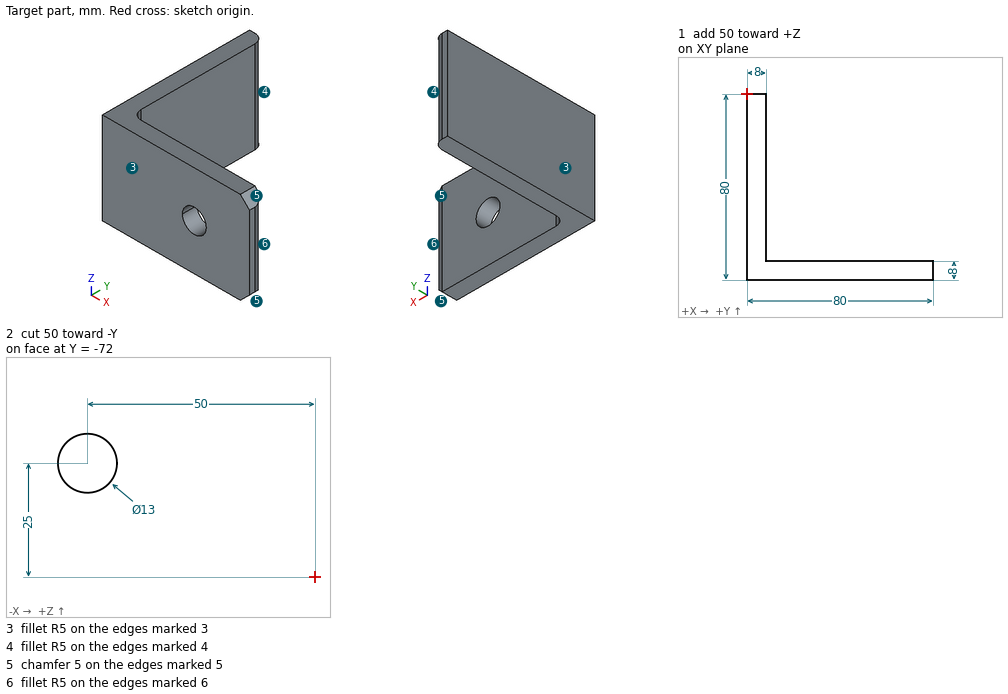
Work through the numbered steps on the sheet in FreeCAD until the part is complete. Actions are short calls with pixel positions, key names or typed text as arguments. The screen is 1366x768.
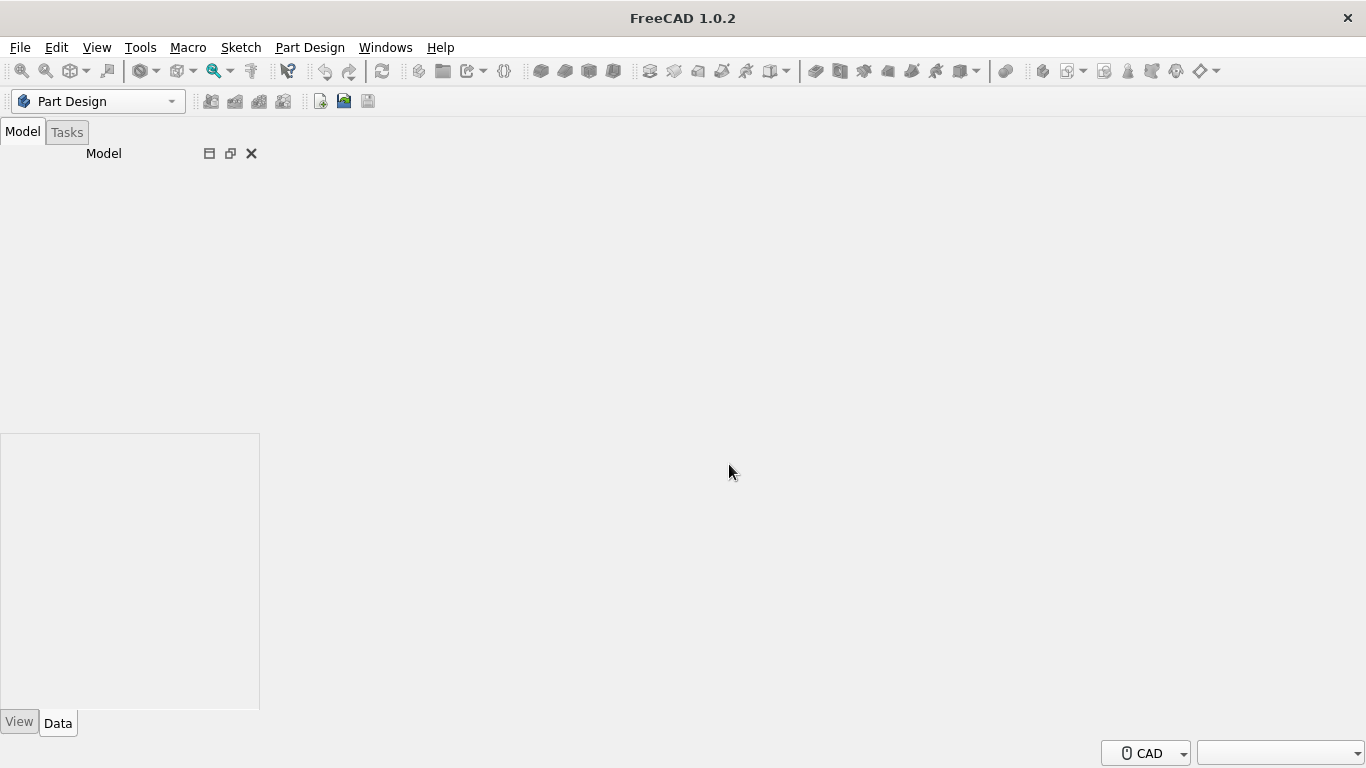
click(320, 102)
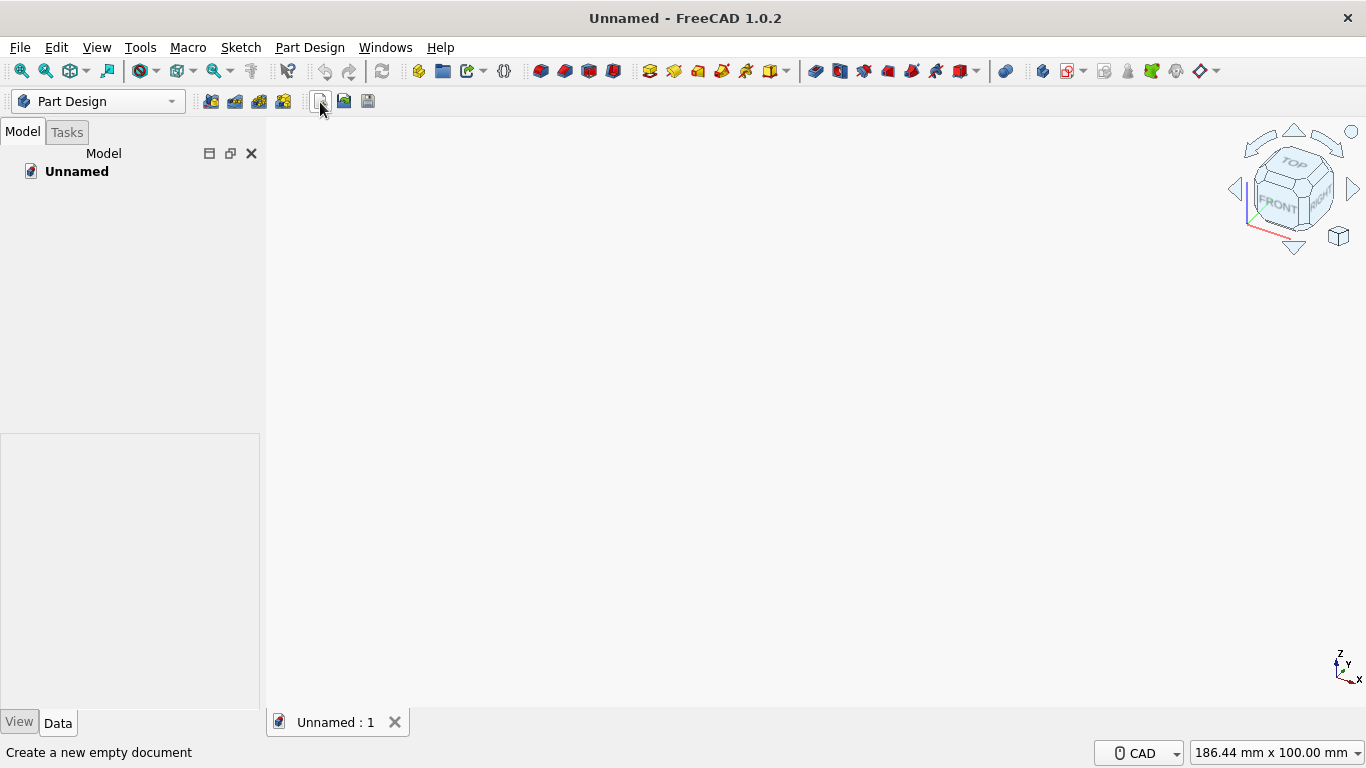
click(1068, 72)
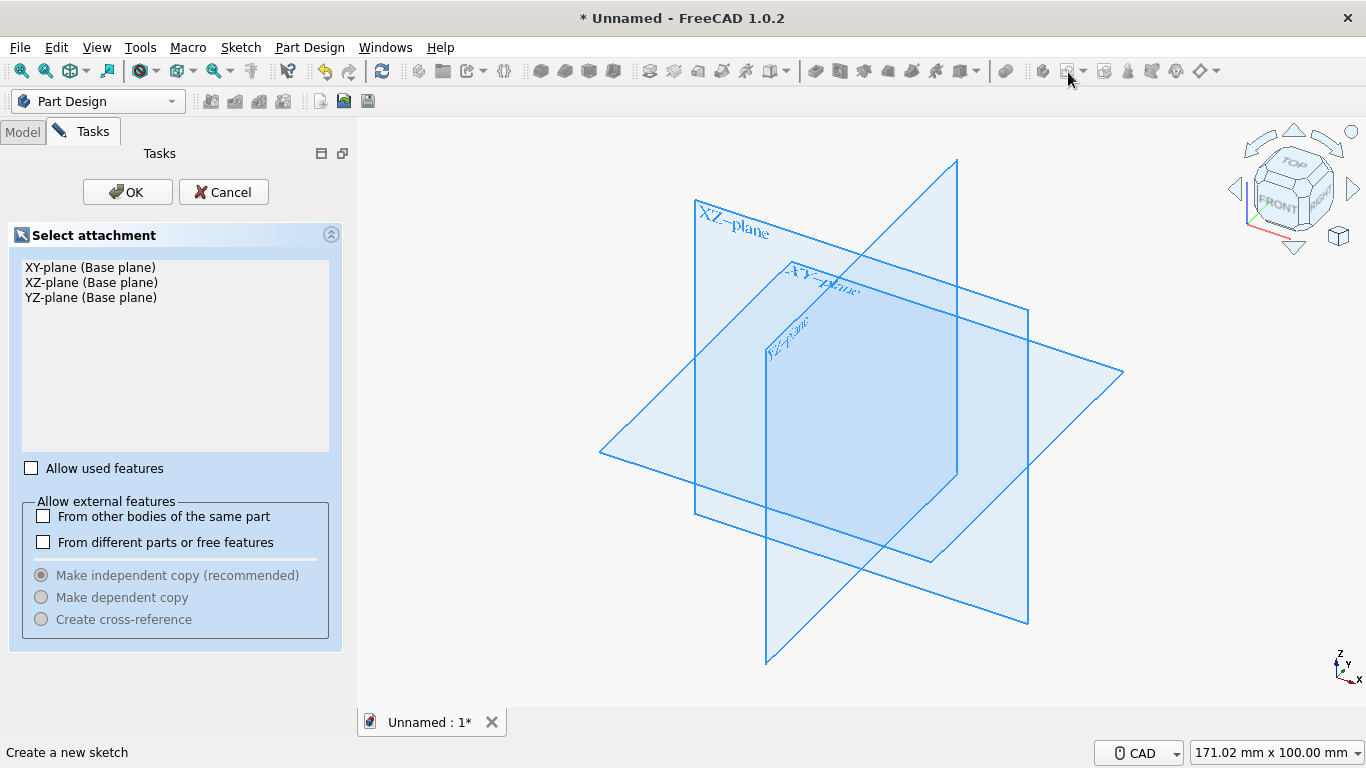
click(82, 268)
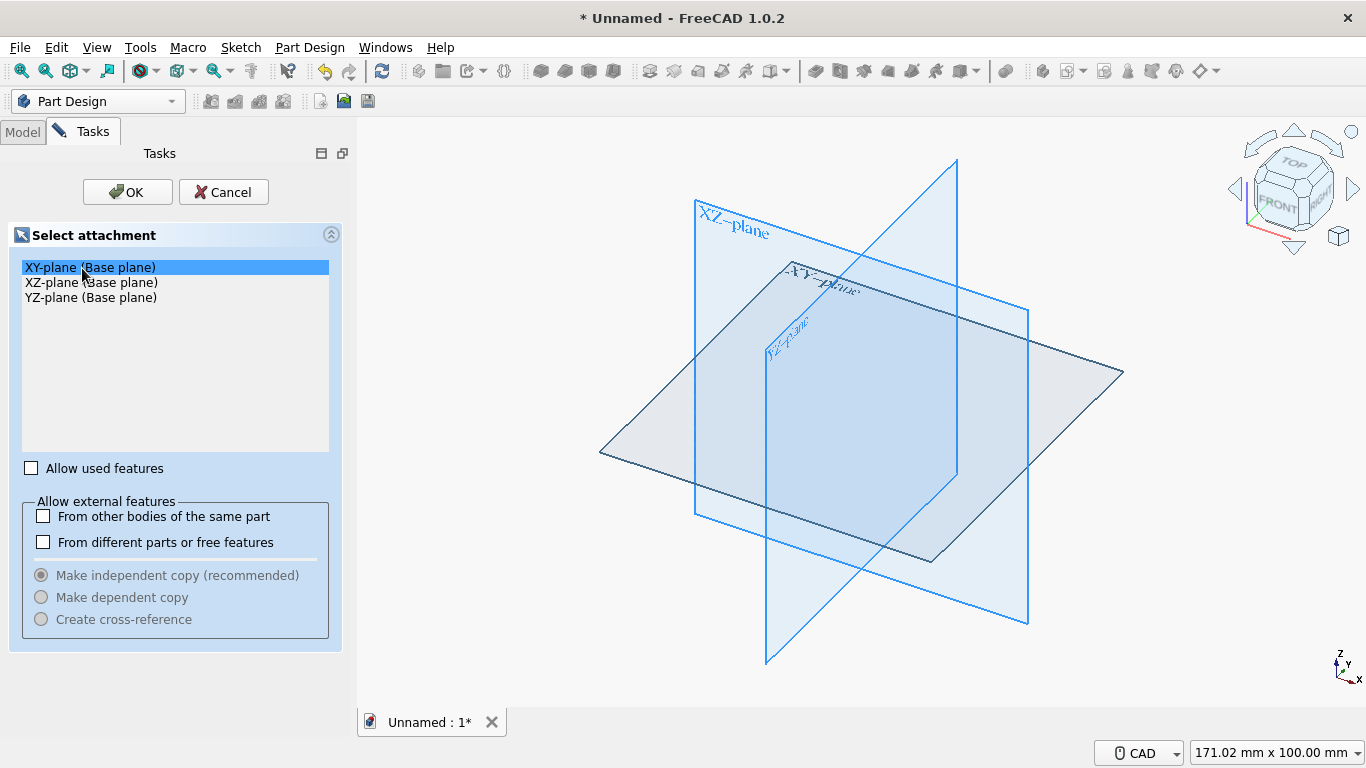
click(128, 192)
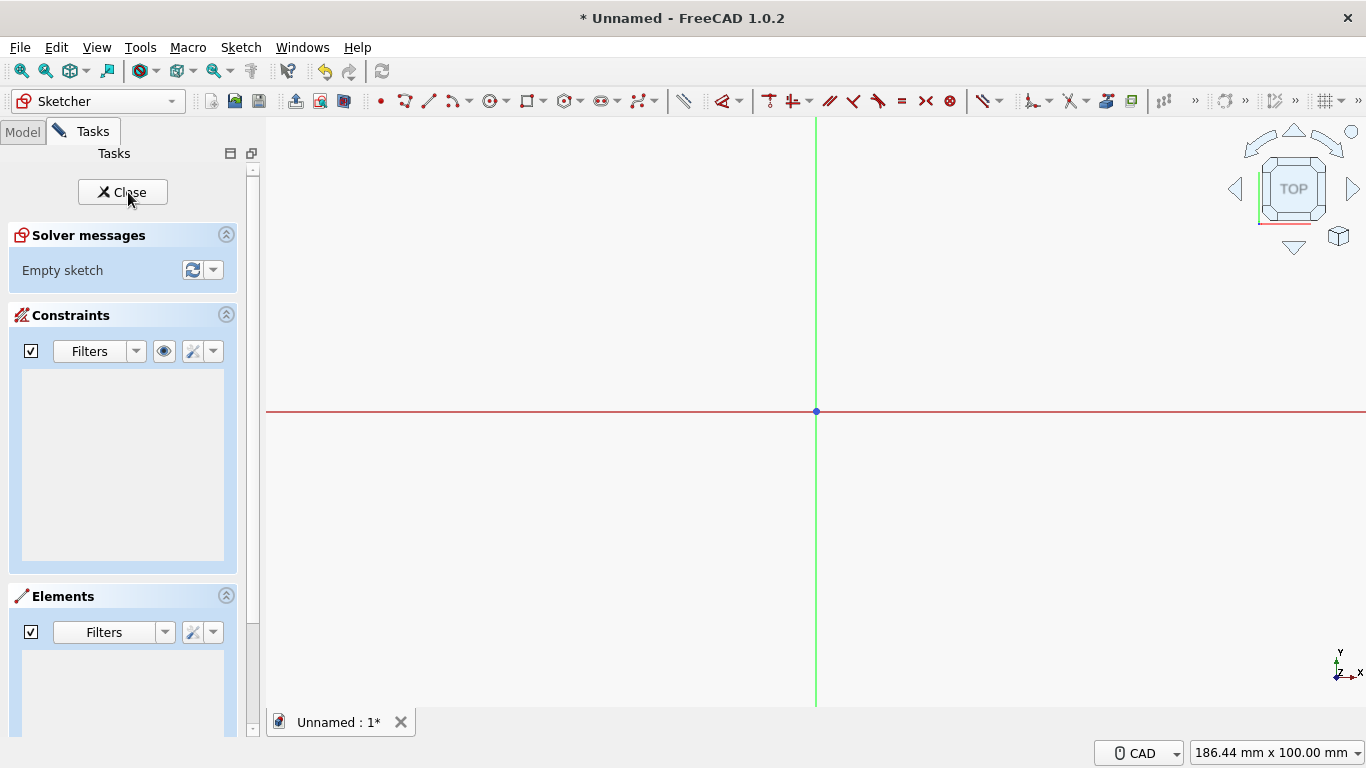
scroll(294, 145, down, 2)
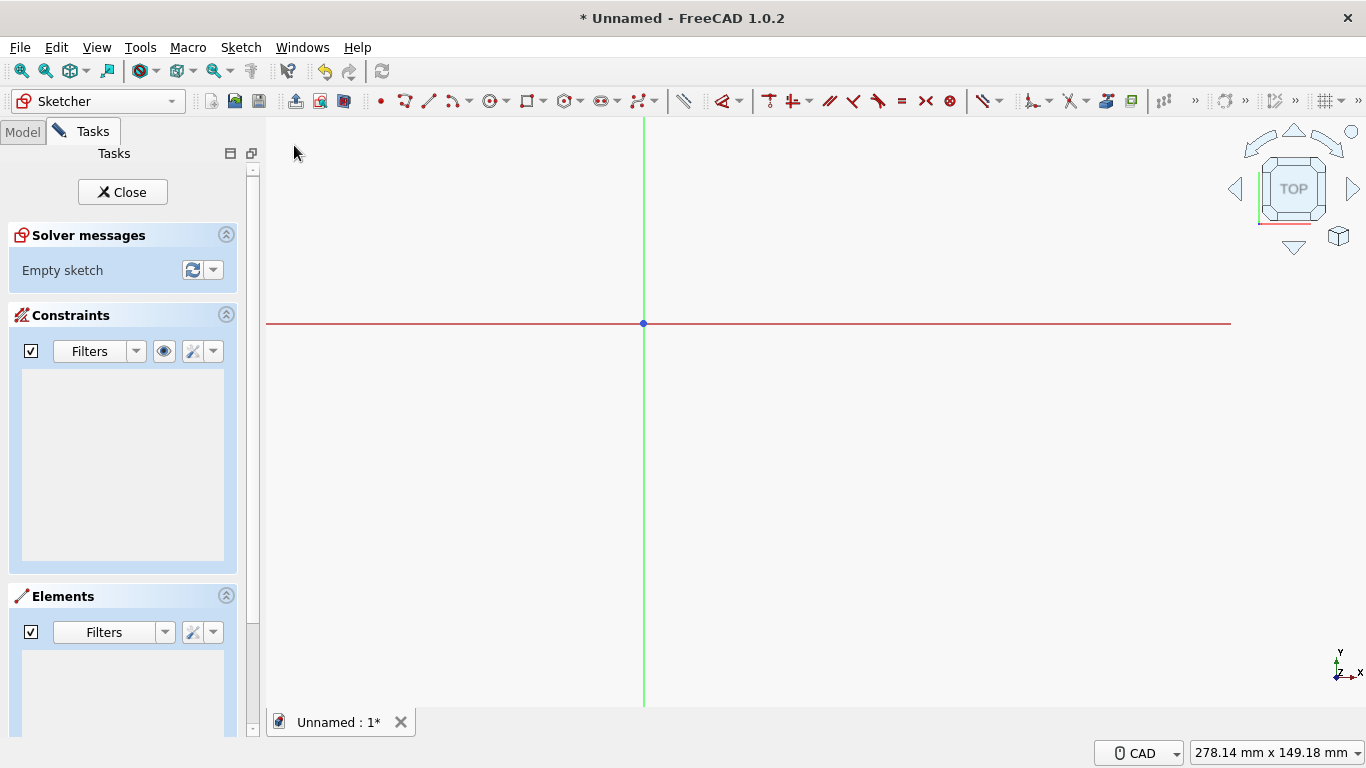
click(406, 102)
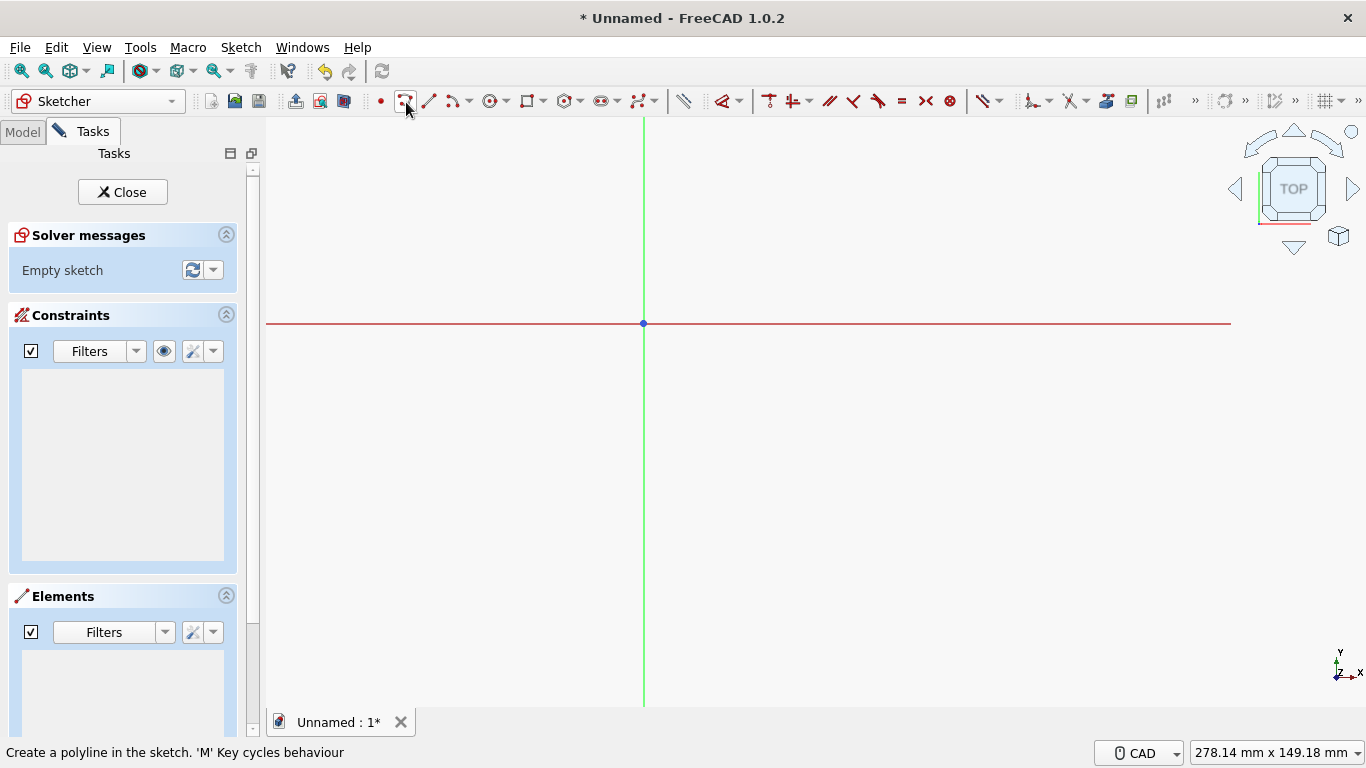
click(644, 324)
click(653, 640)
click(960, 640)
click(960, 609)
click(676, 609)
click(676, 333)
click(644, 324)
key(Escape)
key(Escape)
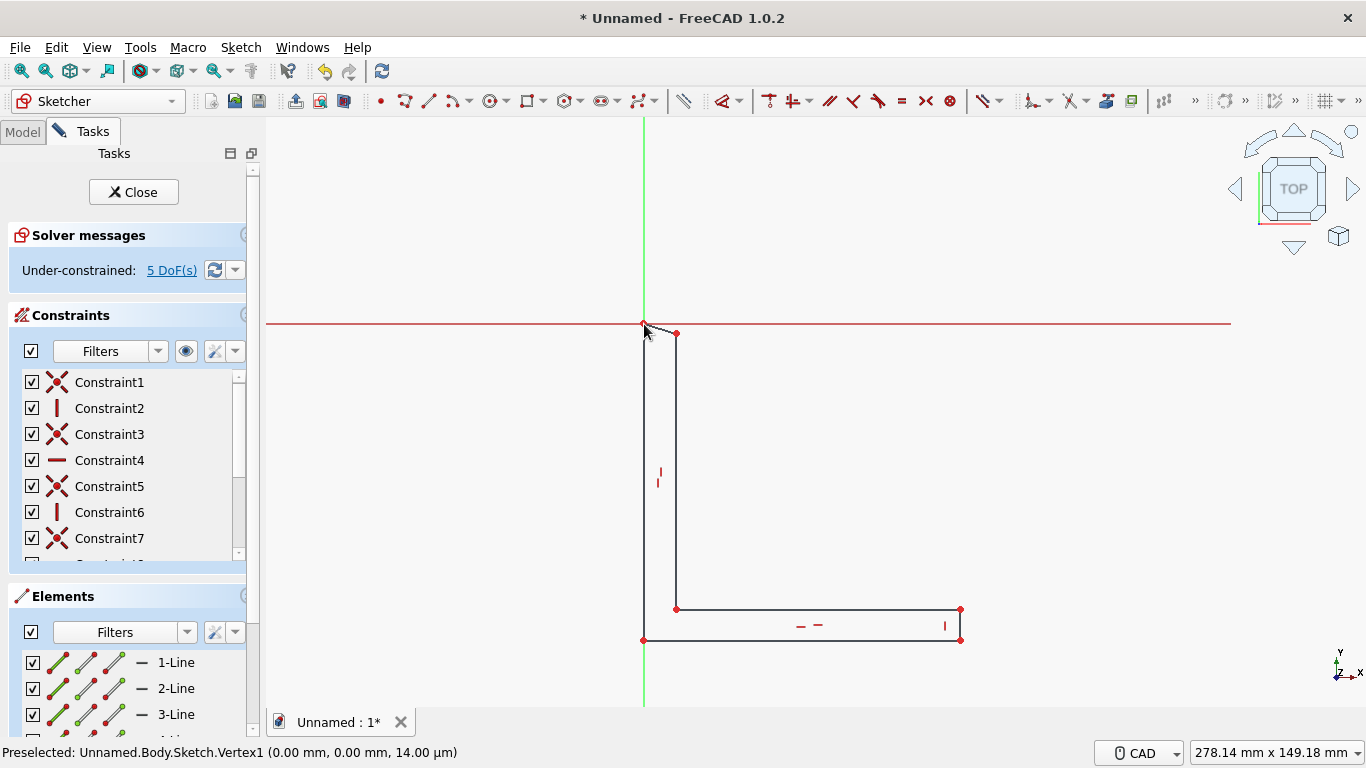
scroll(654, 327, up, 2)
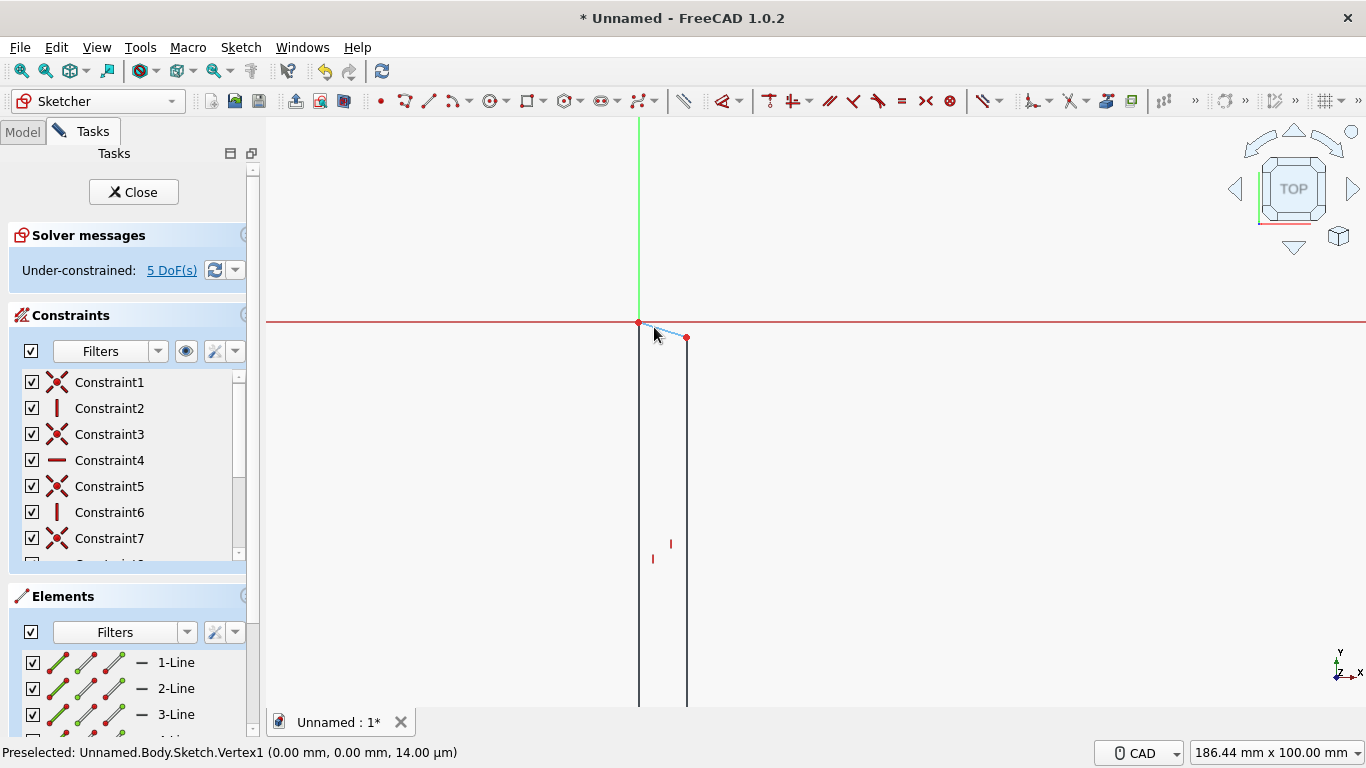
click(653, 327)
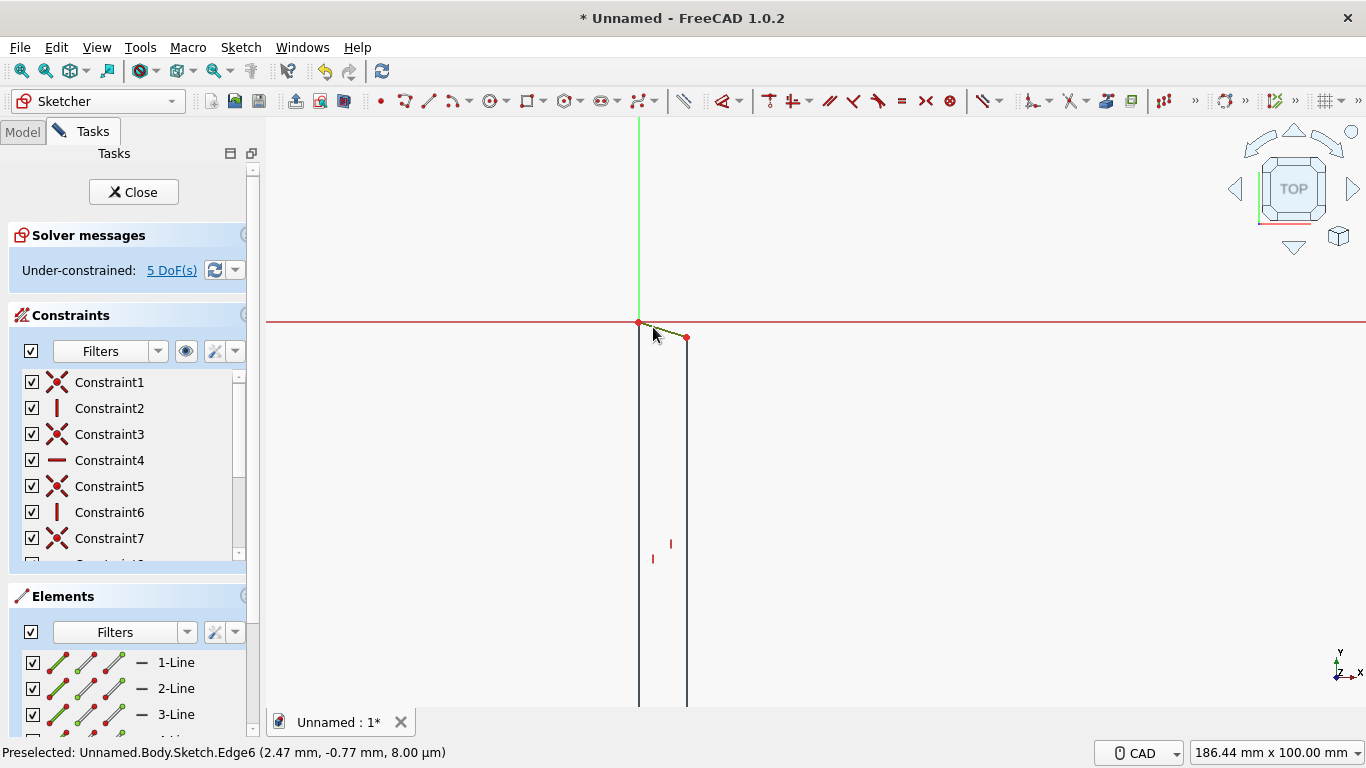
key(h)